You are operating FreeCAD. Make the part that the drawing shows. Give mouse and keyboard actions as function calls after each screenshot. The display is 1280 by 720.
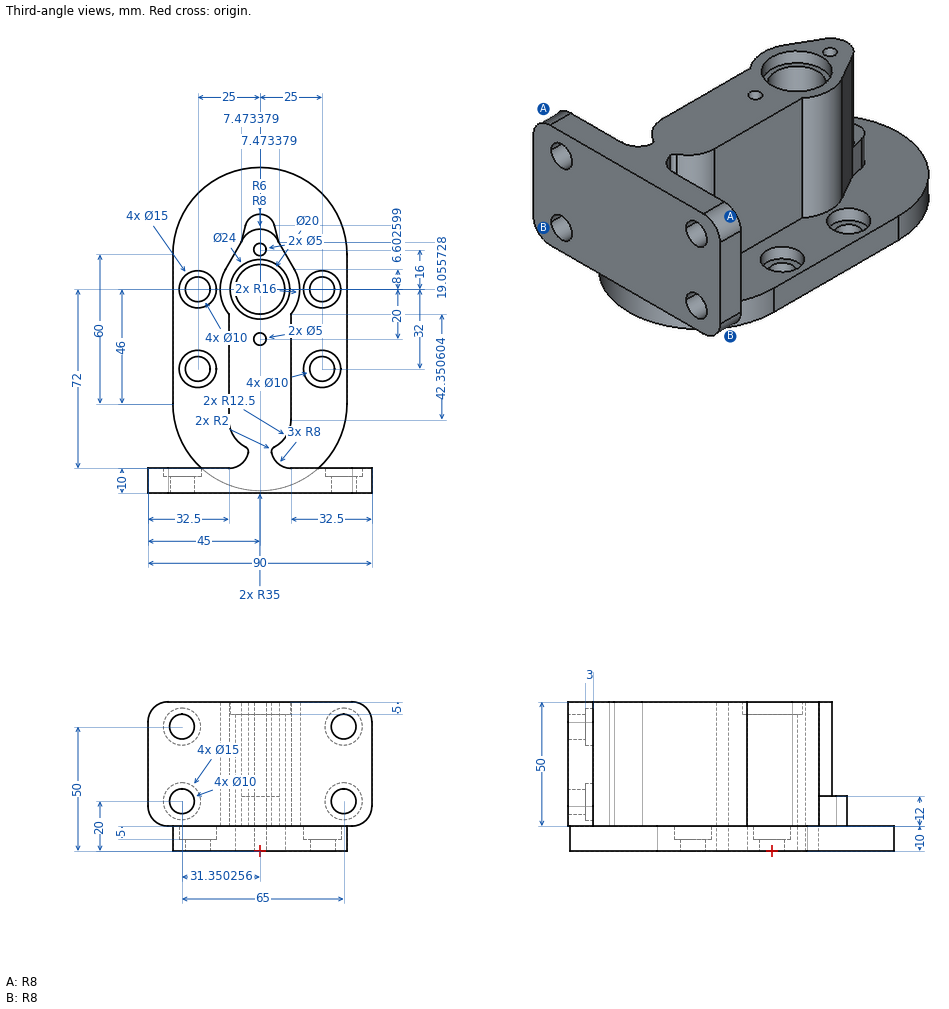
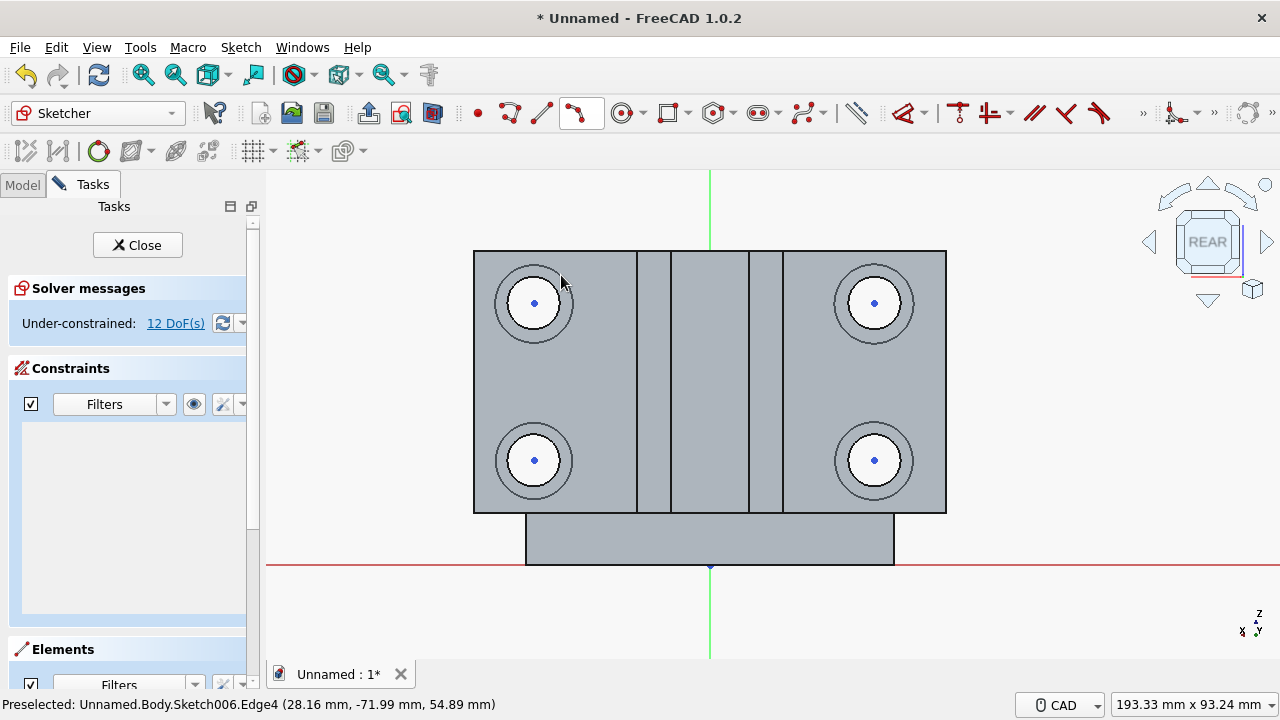
click(901, 433)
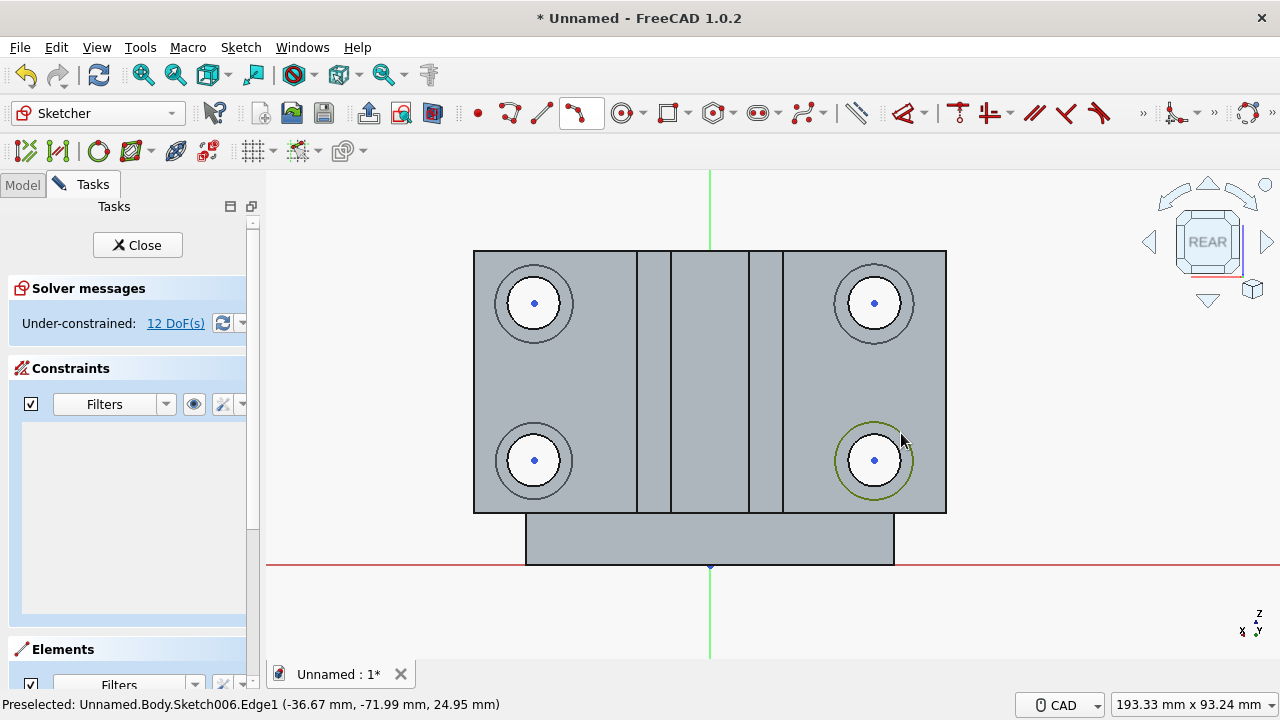
click(902, 276)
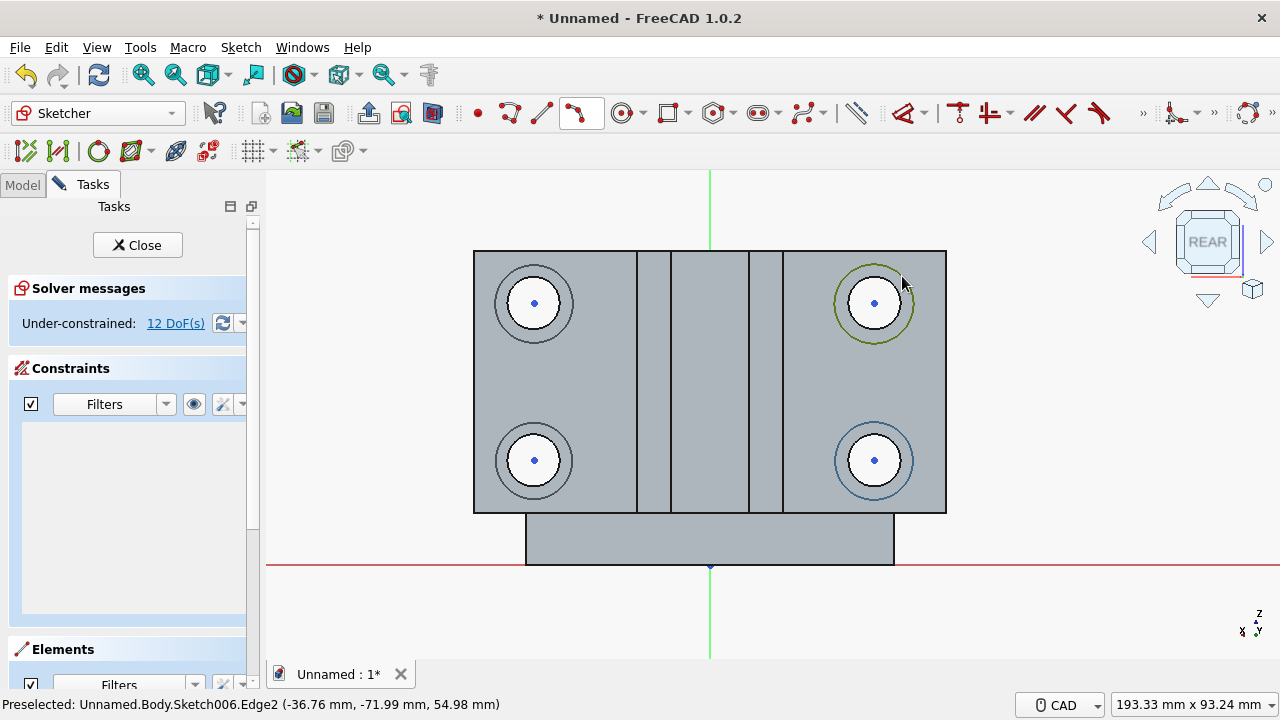
click(561, 434)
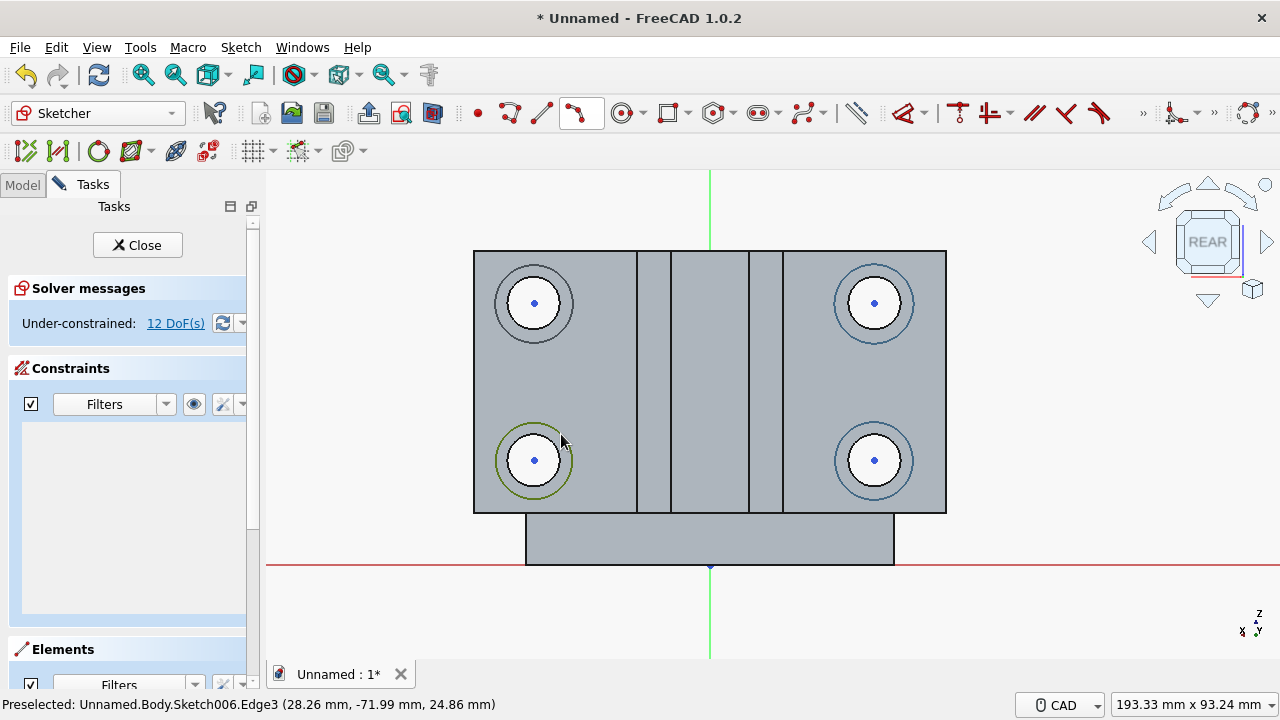
click(561, 276)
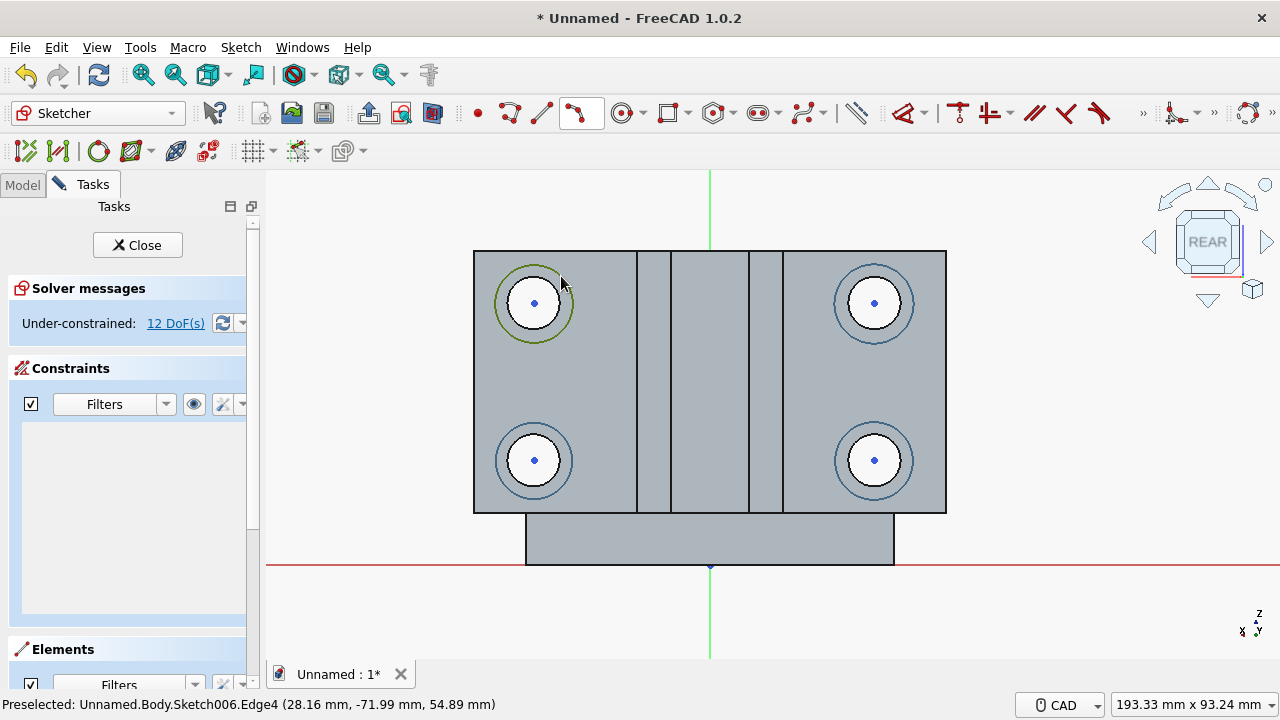
key(e)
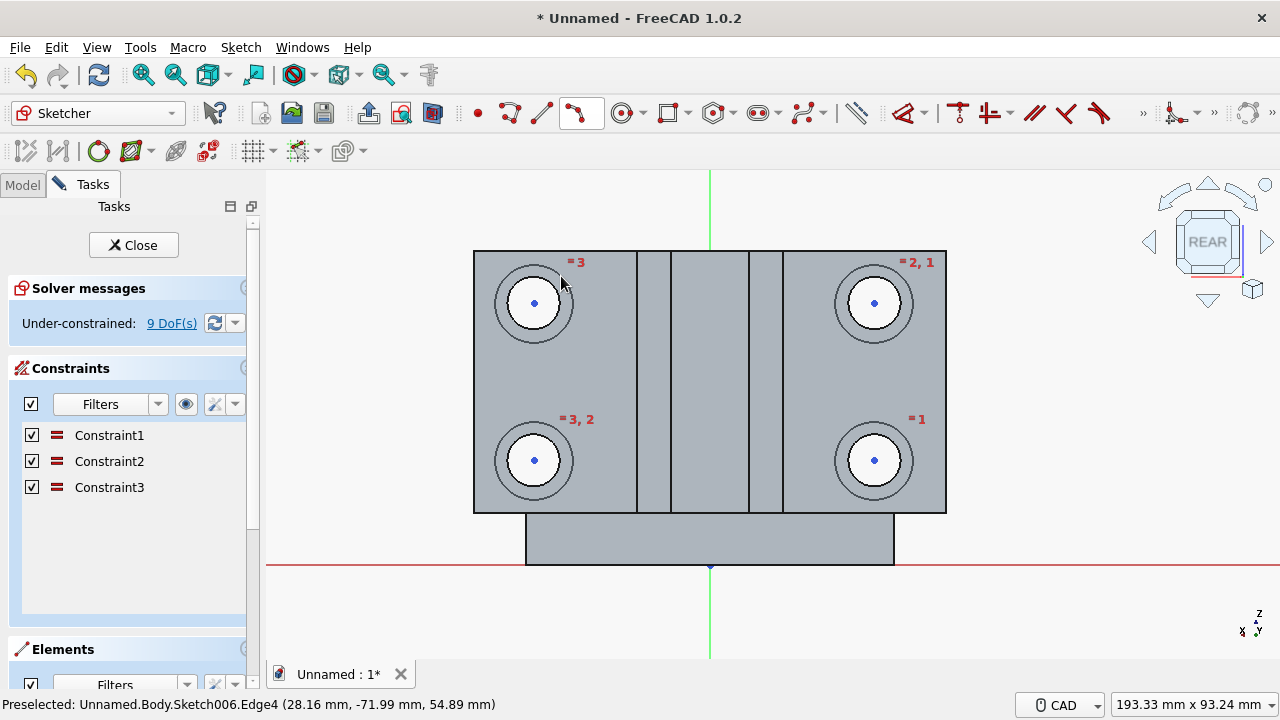
click(904, 114)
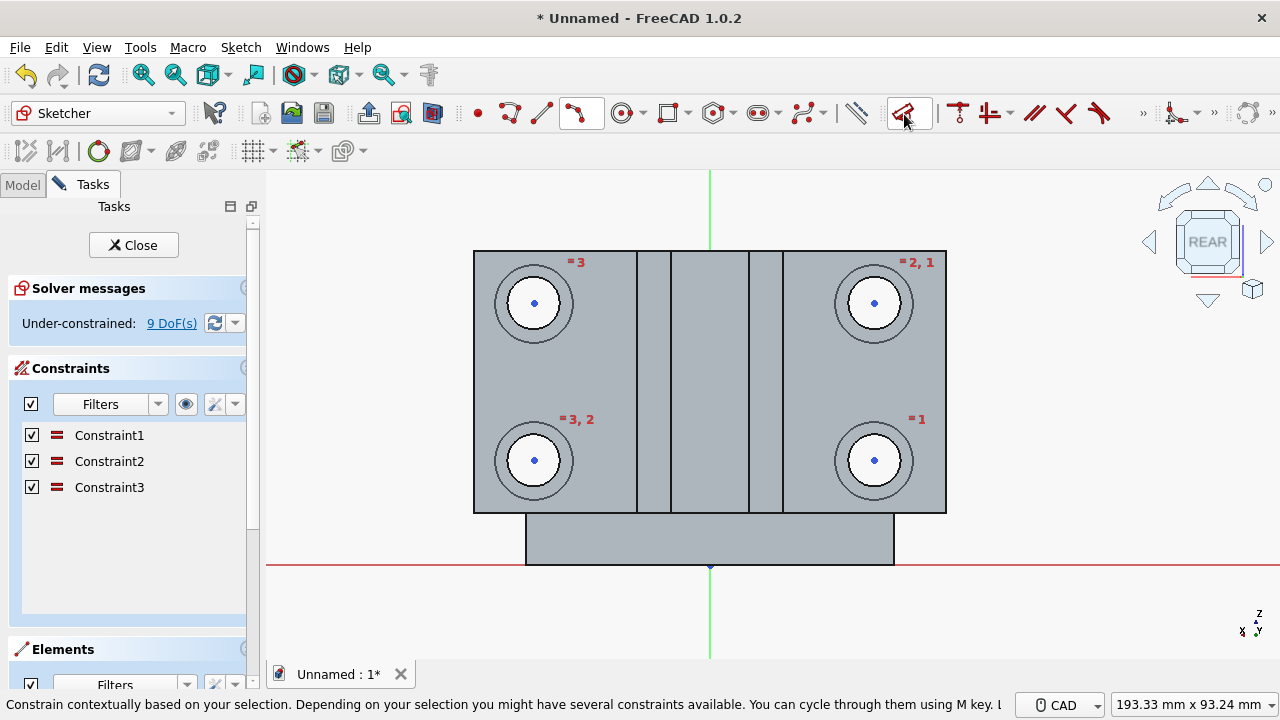
click(901, 433)
click(923, 410)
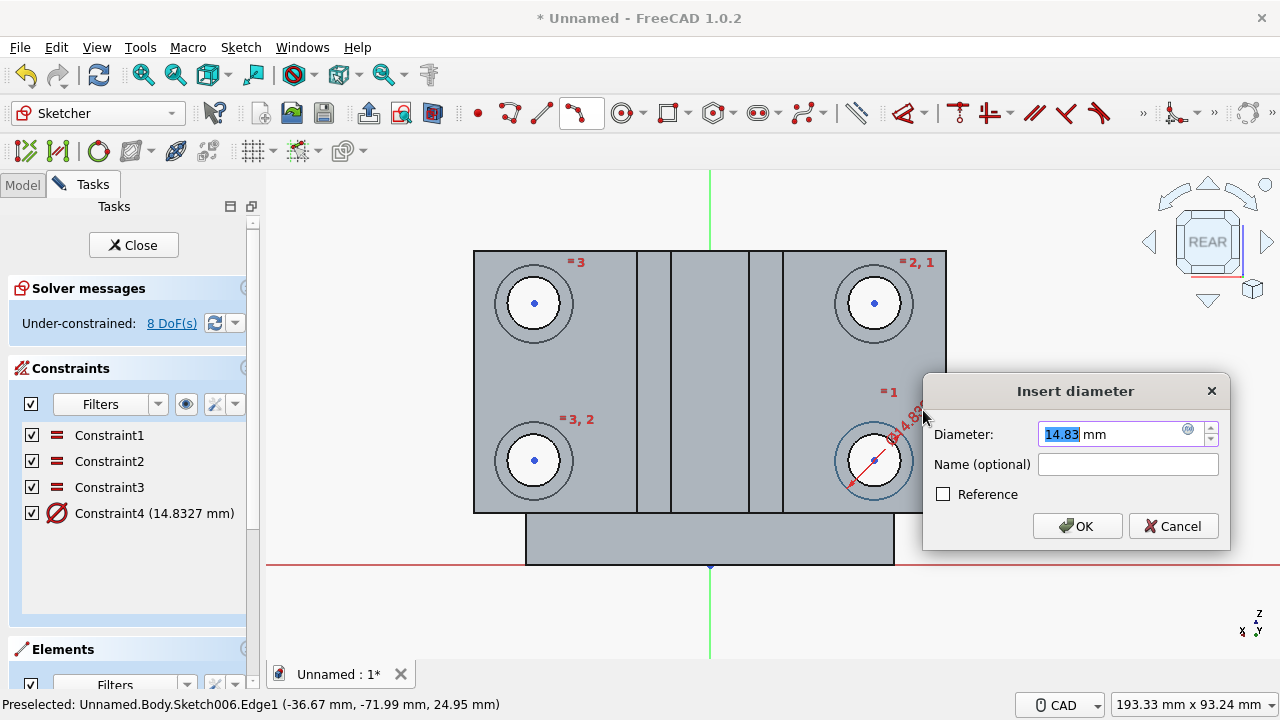
text(15)
key(Return)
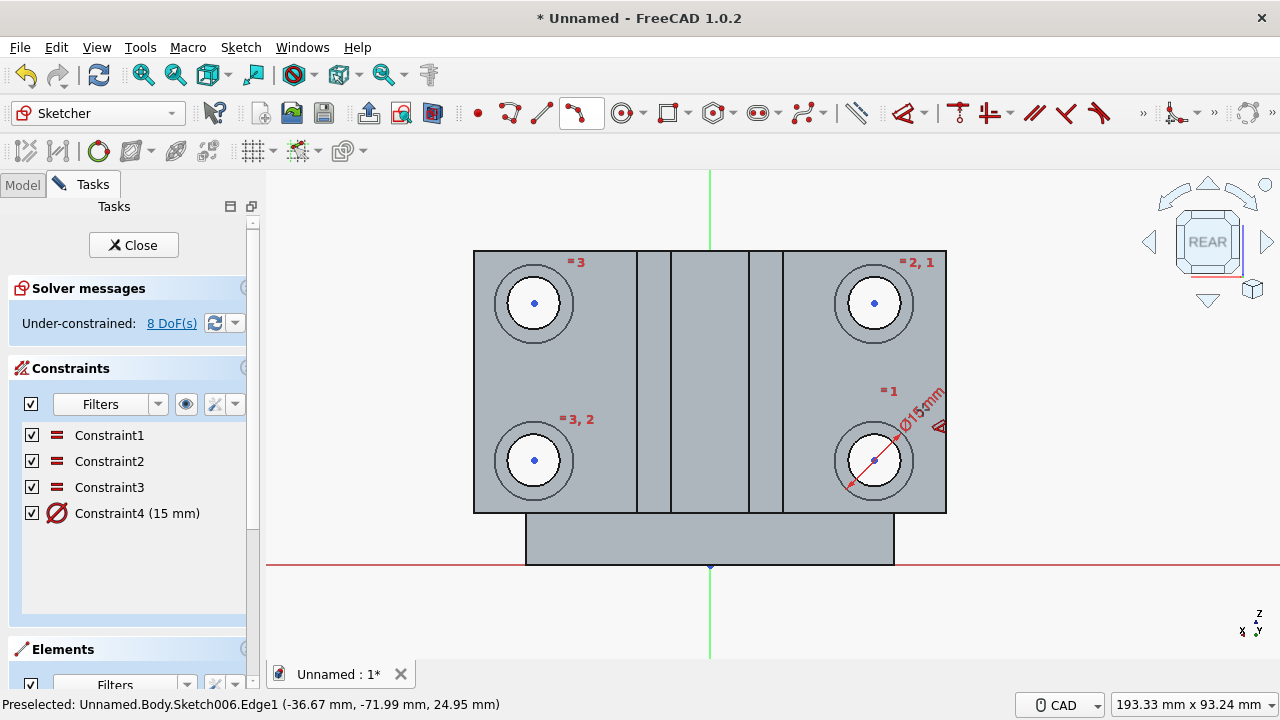
click(874, 461)
click(908, 513)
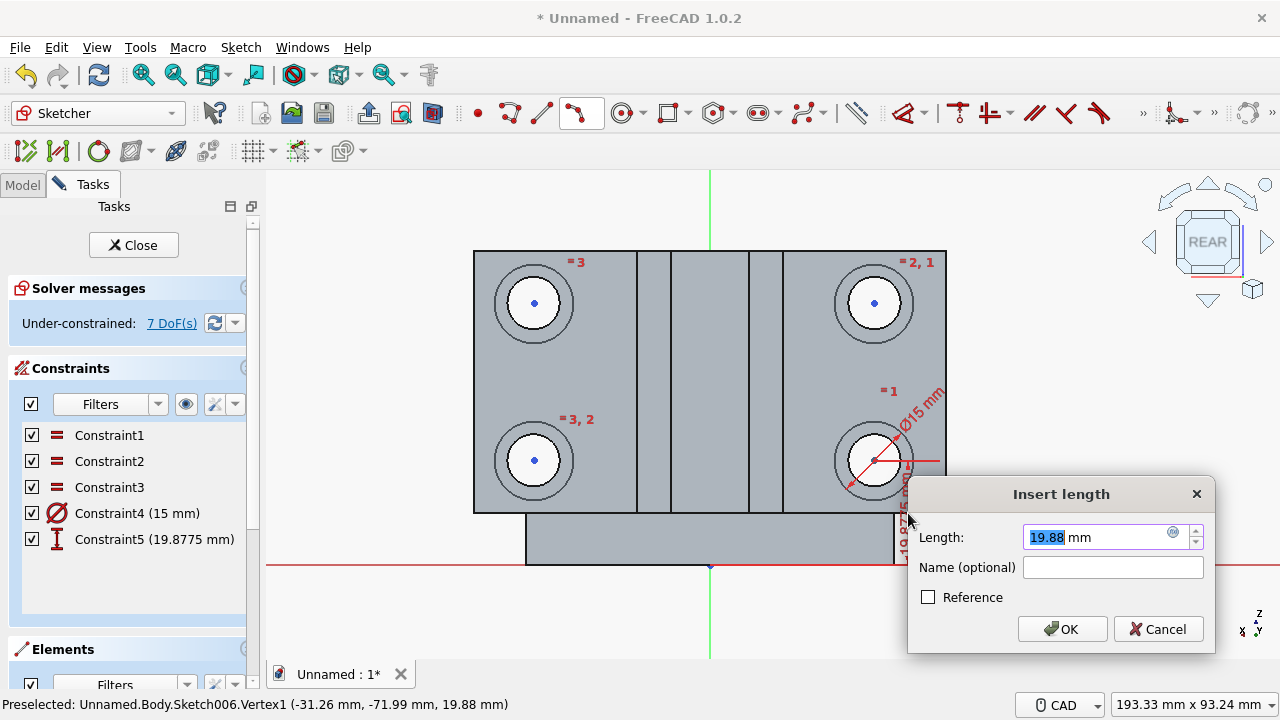
text(20)
key(Return)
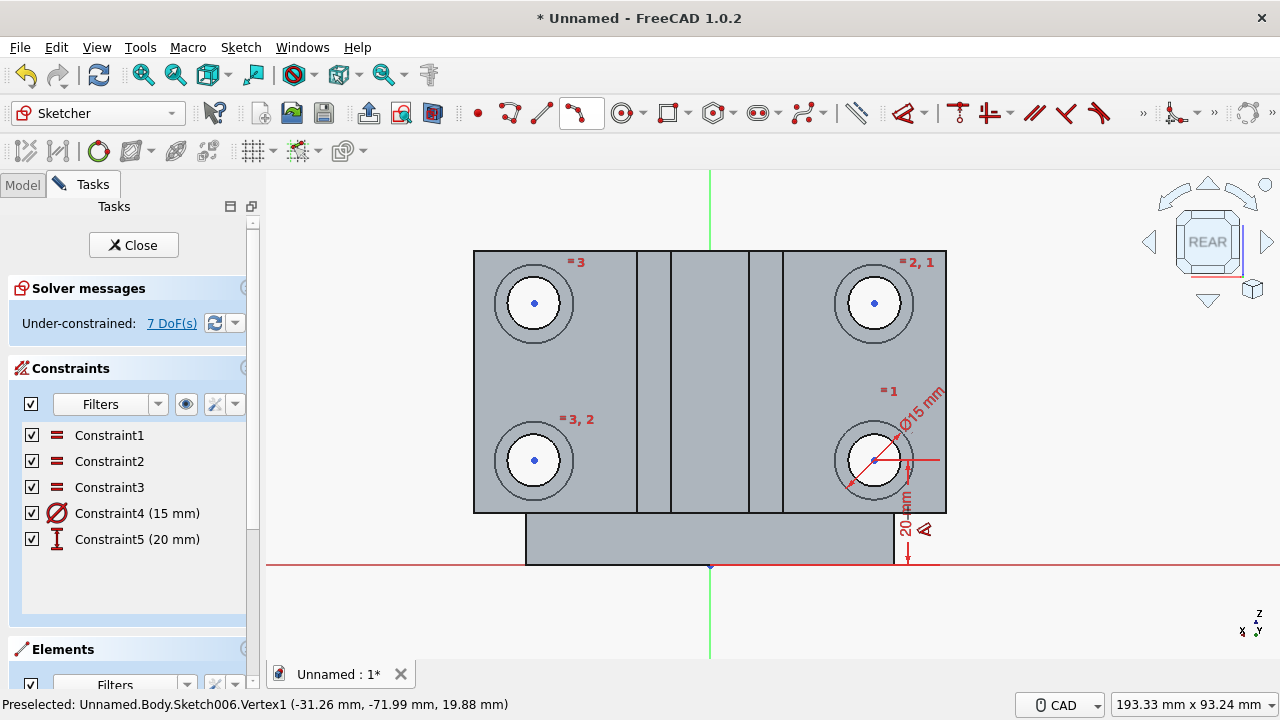
click(874, 304)
click(908, 375)